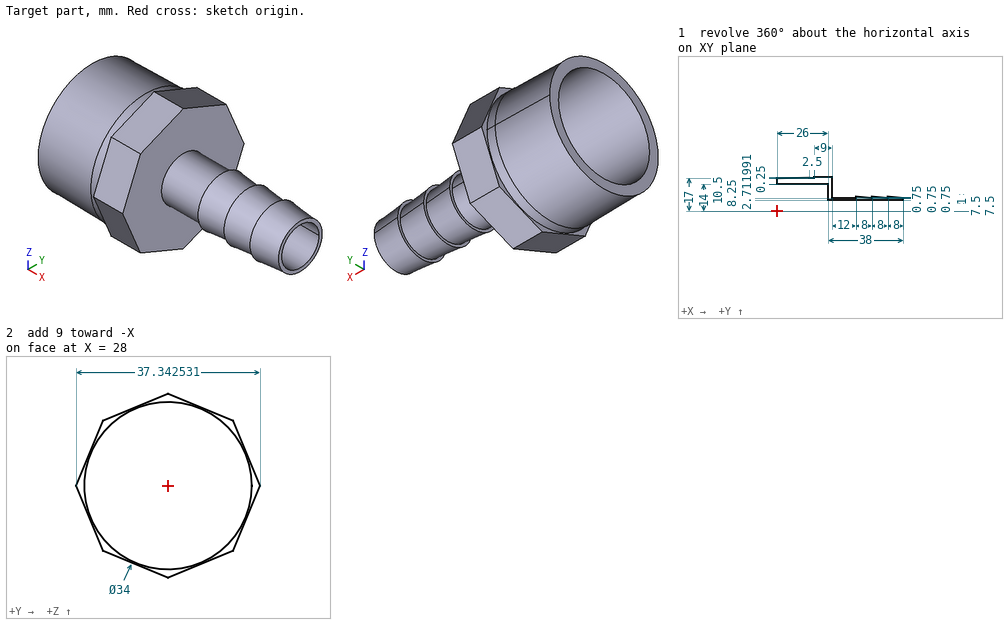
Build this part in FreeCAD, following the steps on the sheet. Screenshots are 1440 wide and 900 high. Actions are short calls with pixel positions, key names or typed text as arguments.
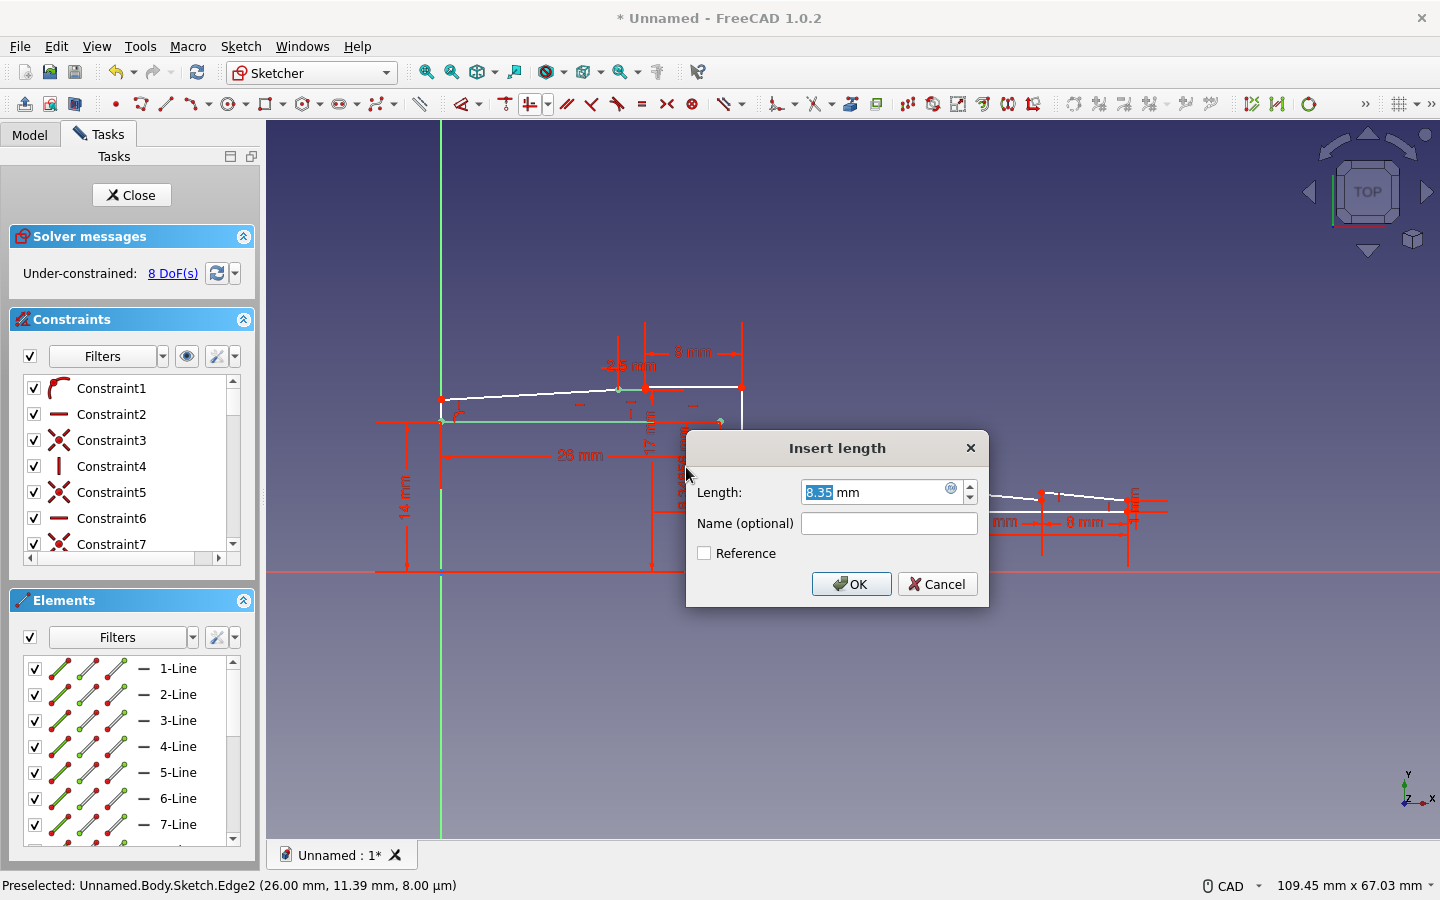
text(8.25)
key(Return)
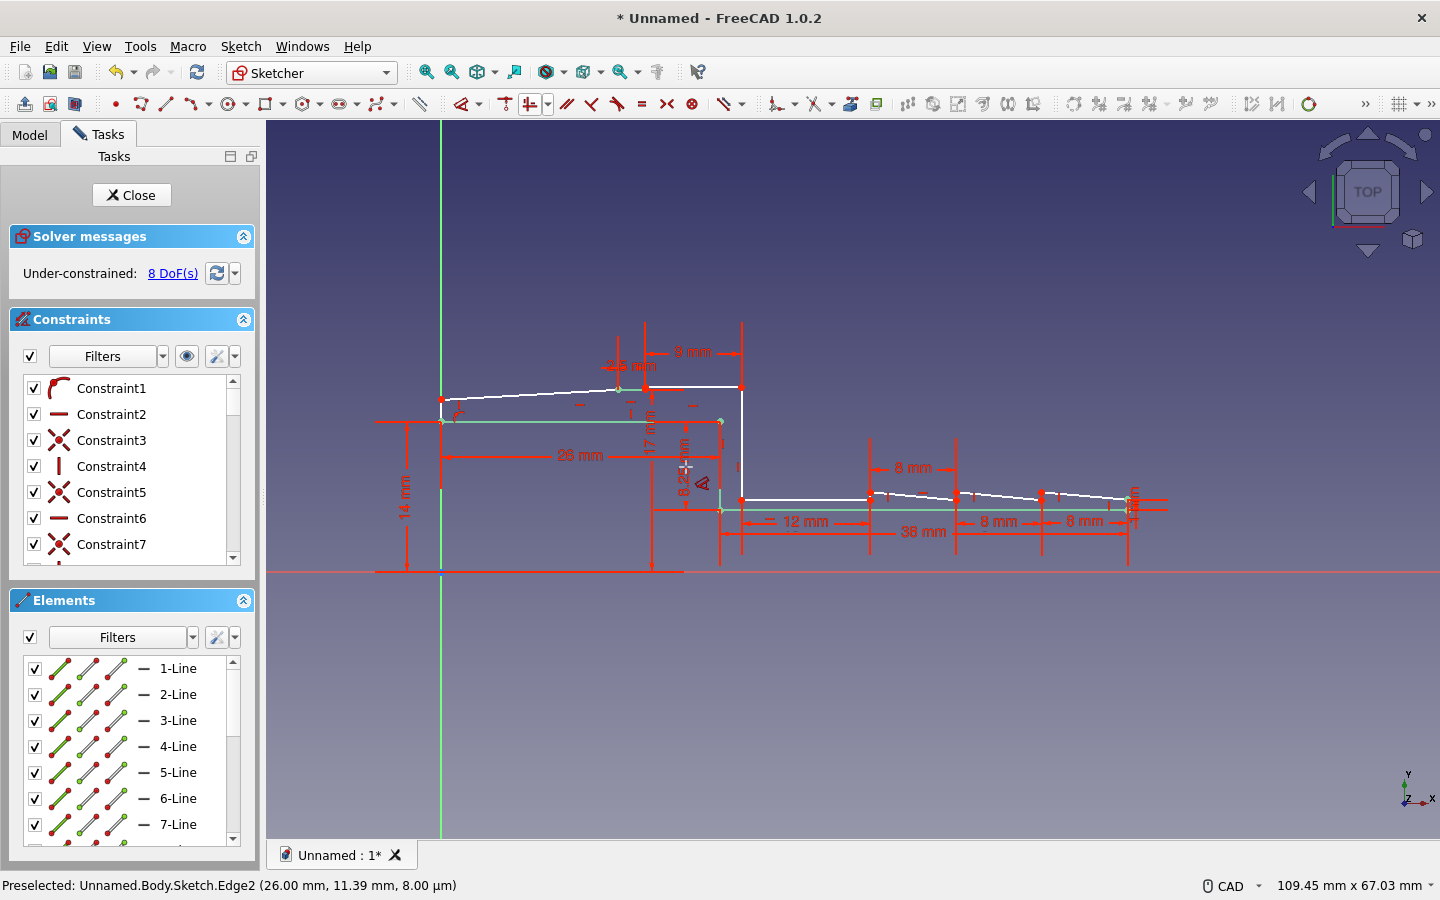
scroll(1042, 496, up, 8)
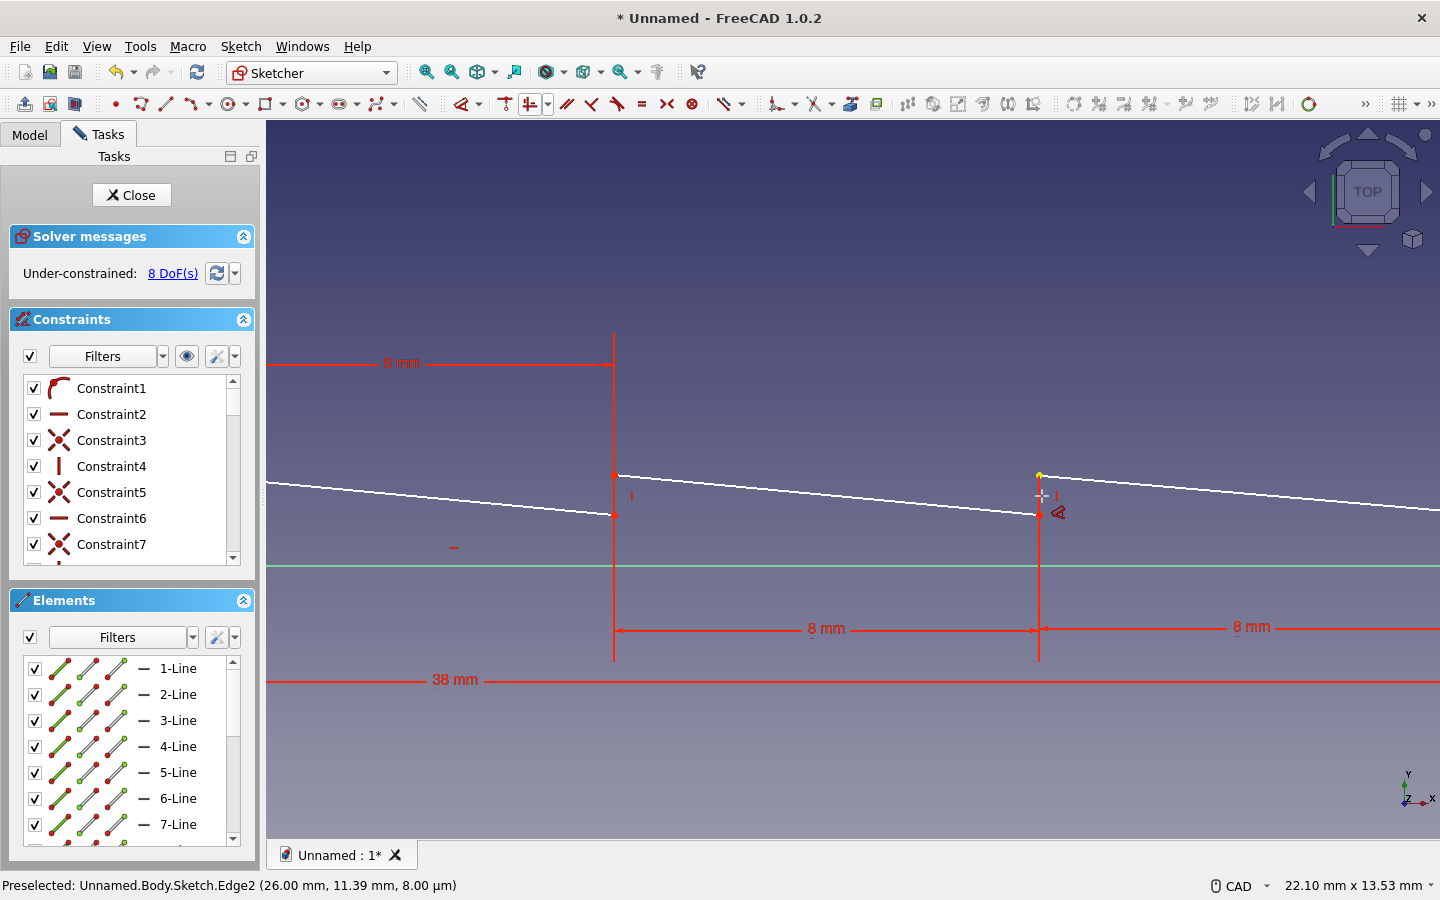
click(1039, 495)
click(1073, 495)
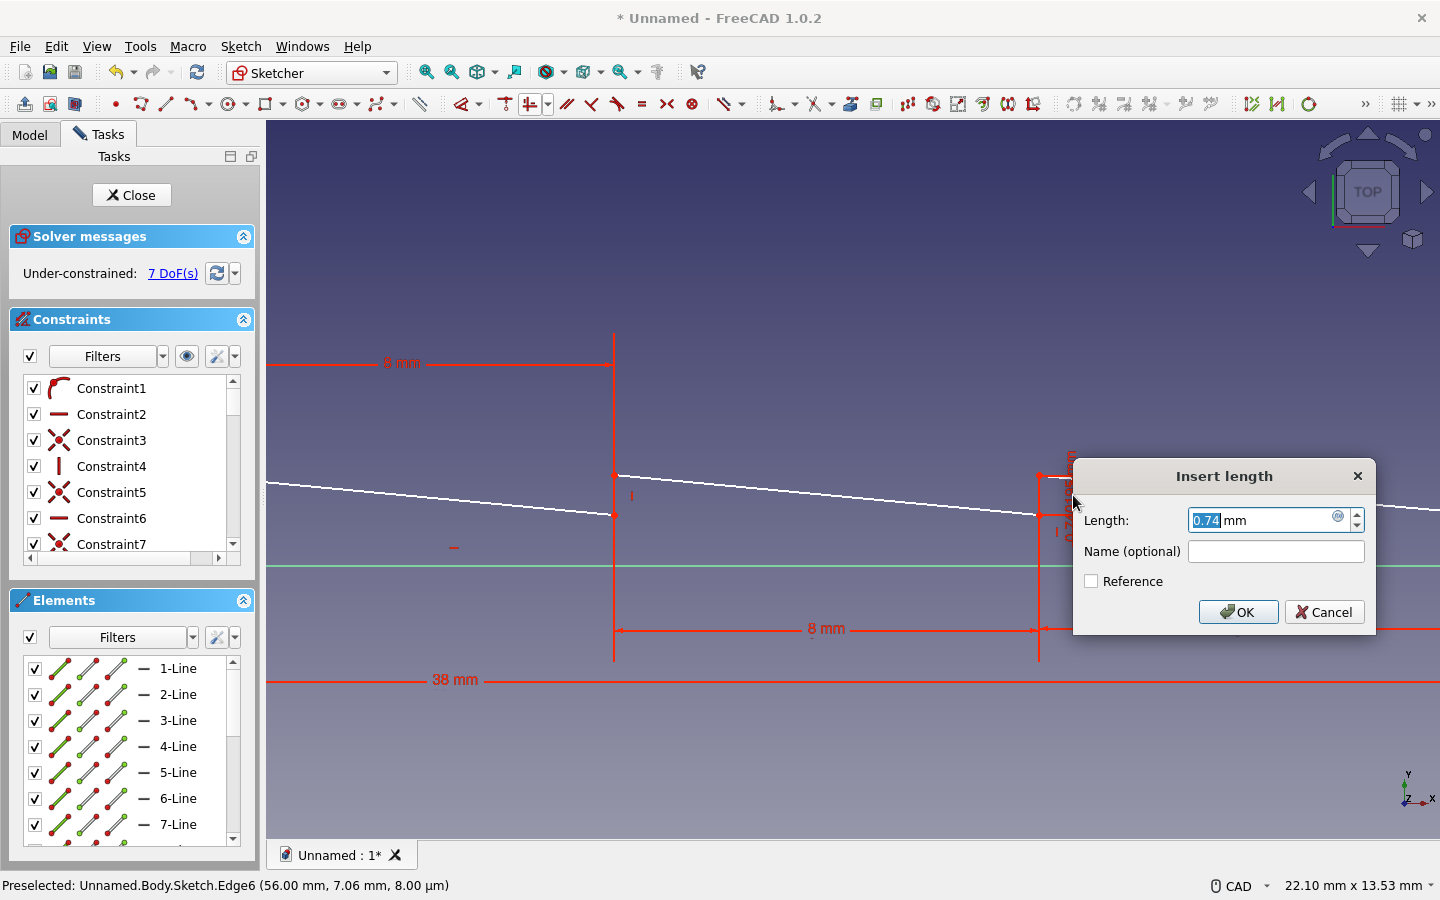
text(0.75)
key(Return)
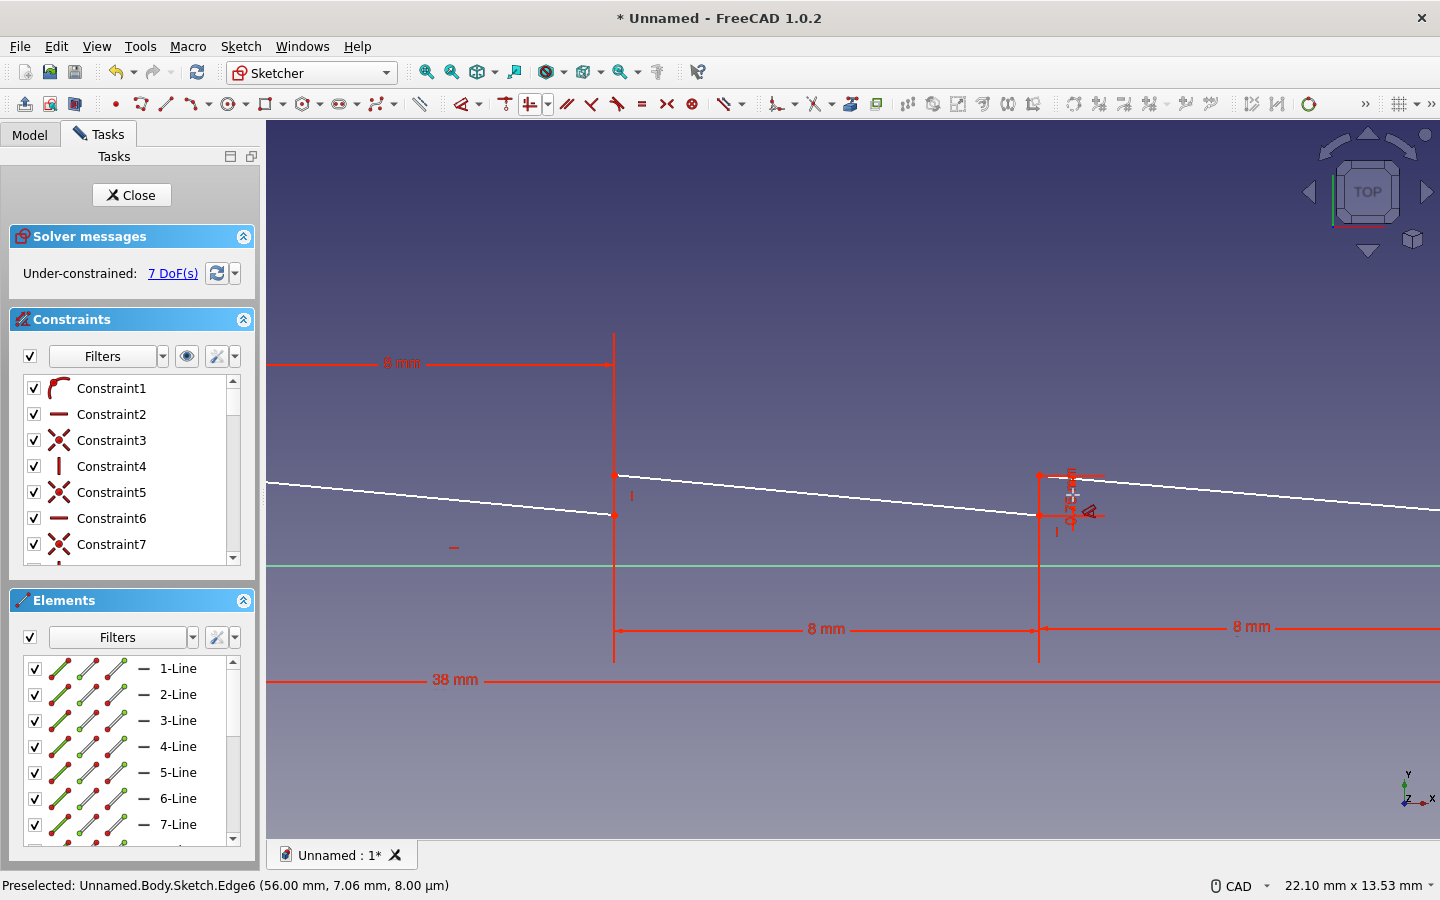
click(614, 487)
click(648, 495)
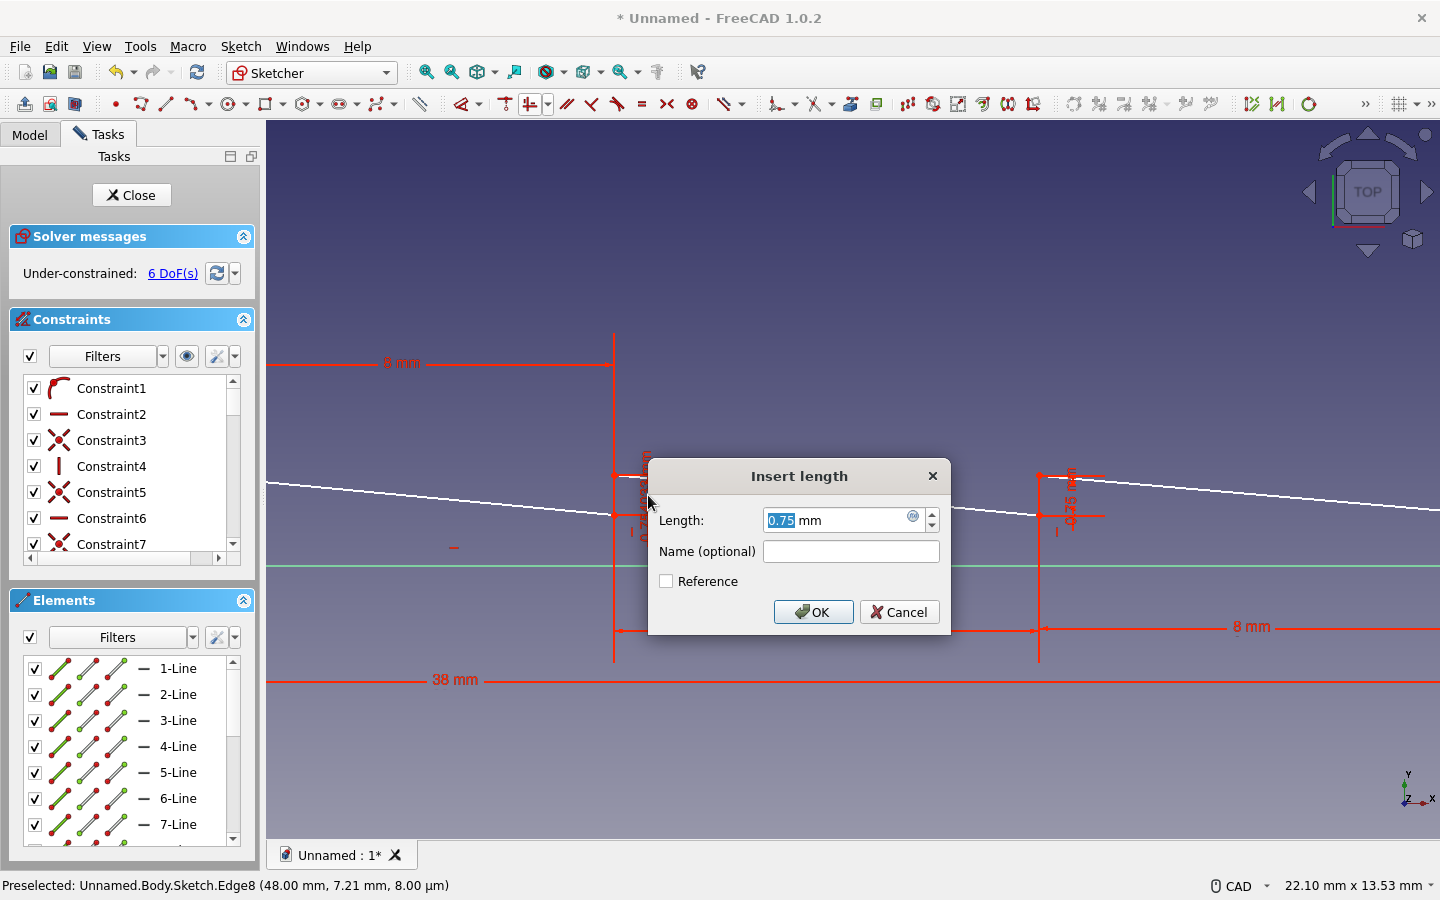
text(0.75)
key(Return)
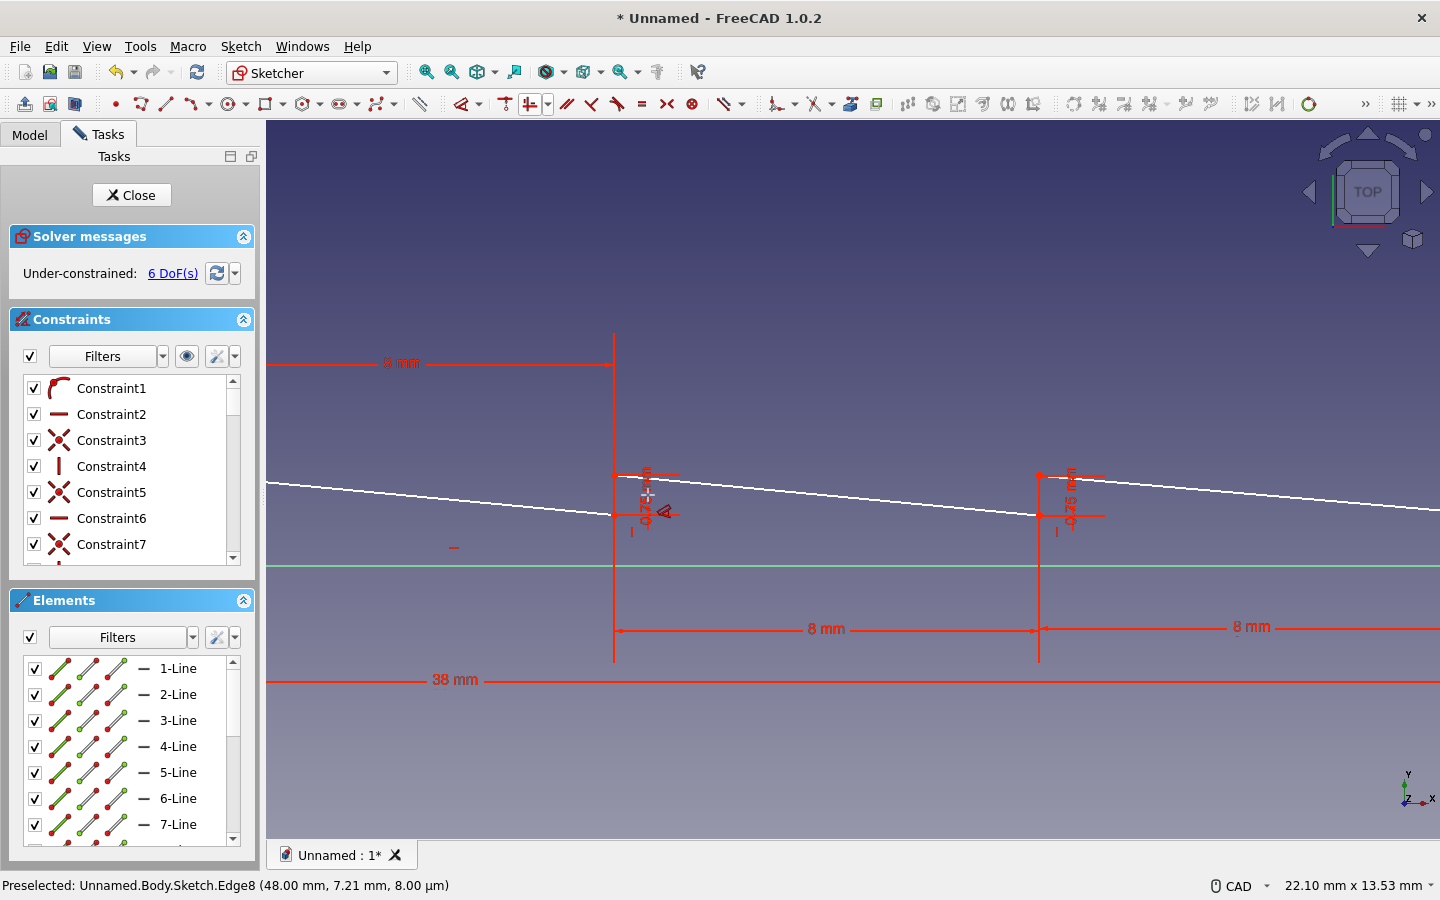
scroll(1043, 496, down, 8)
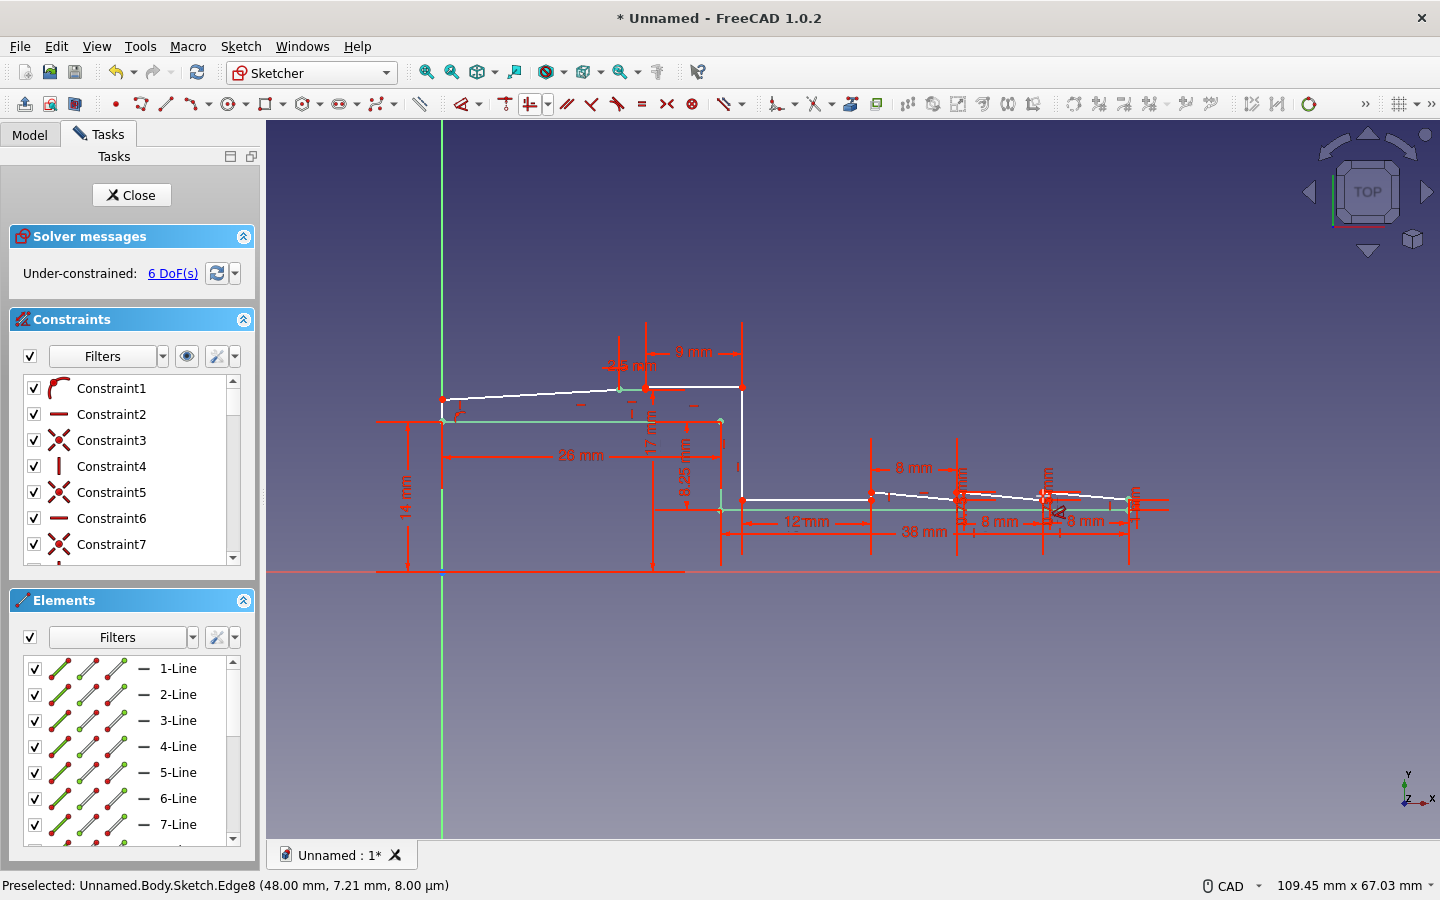
scroll(871, 495, up, 9)